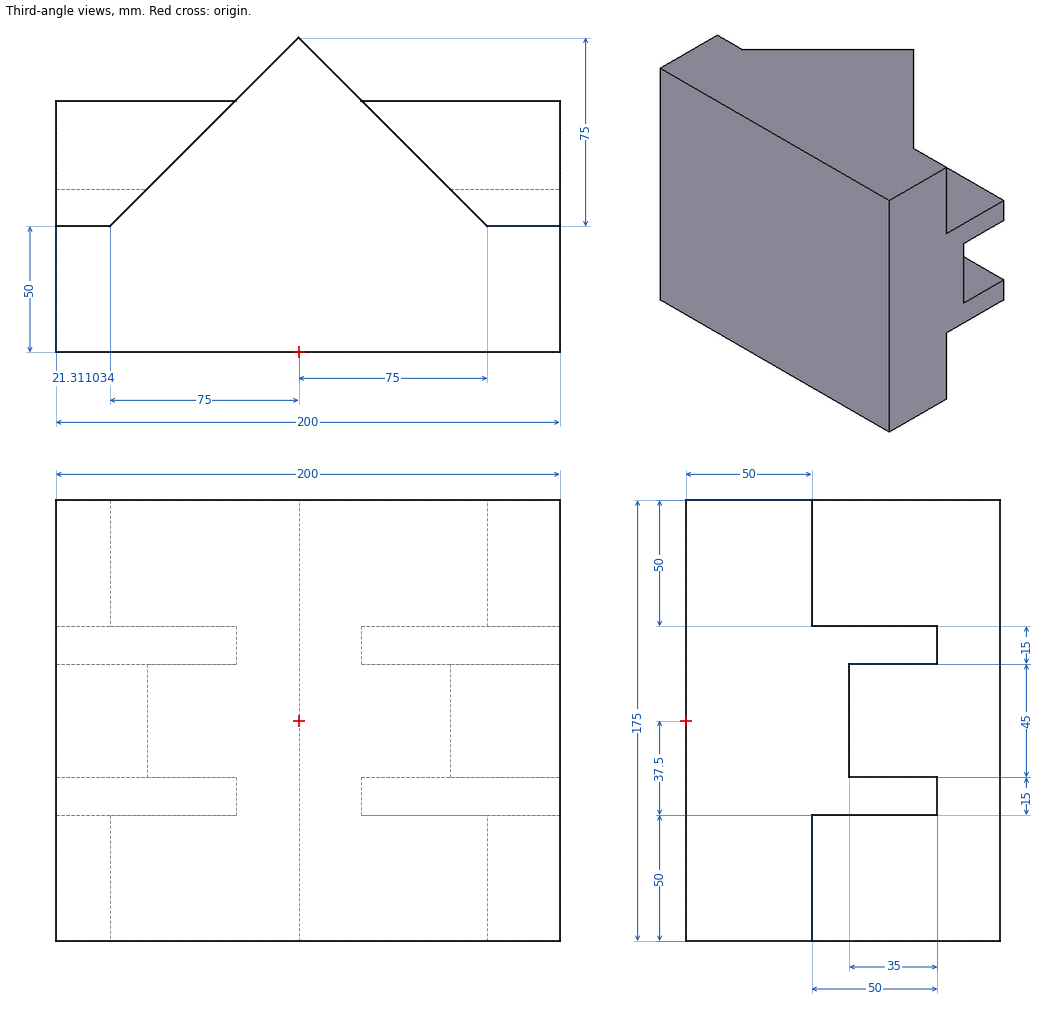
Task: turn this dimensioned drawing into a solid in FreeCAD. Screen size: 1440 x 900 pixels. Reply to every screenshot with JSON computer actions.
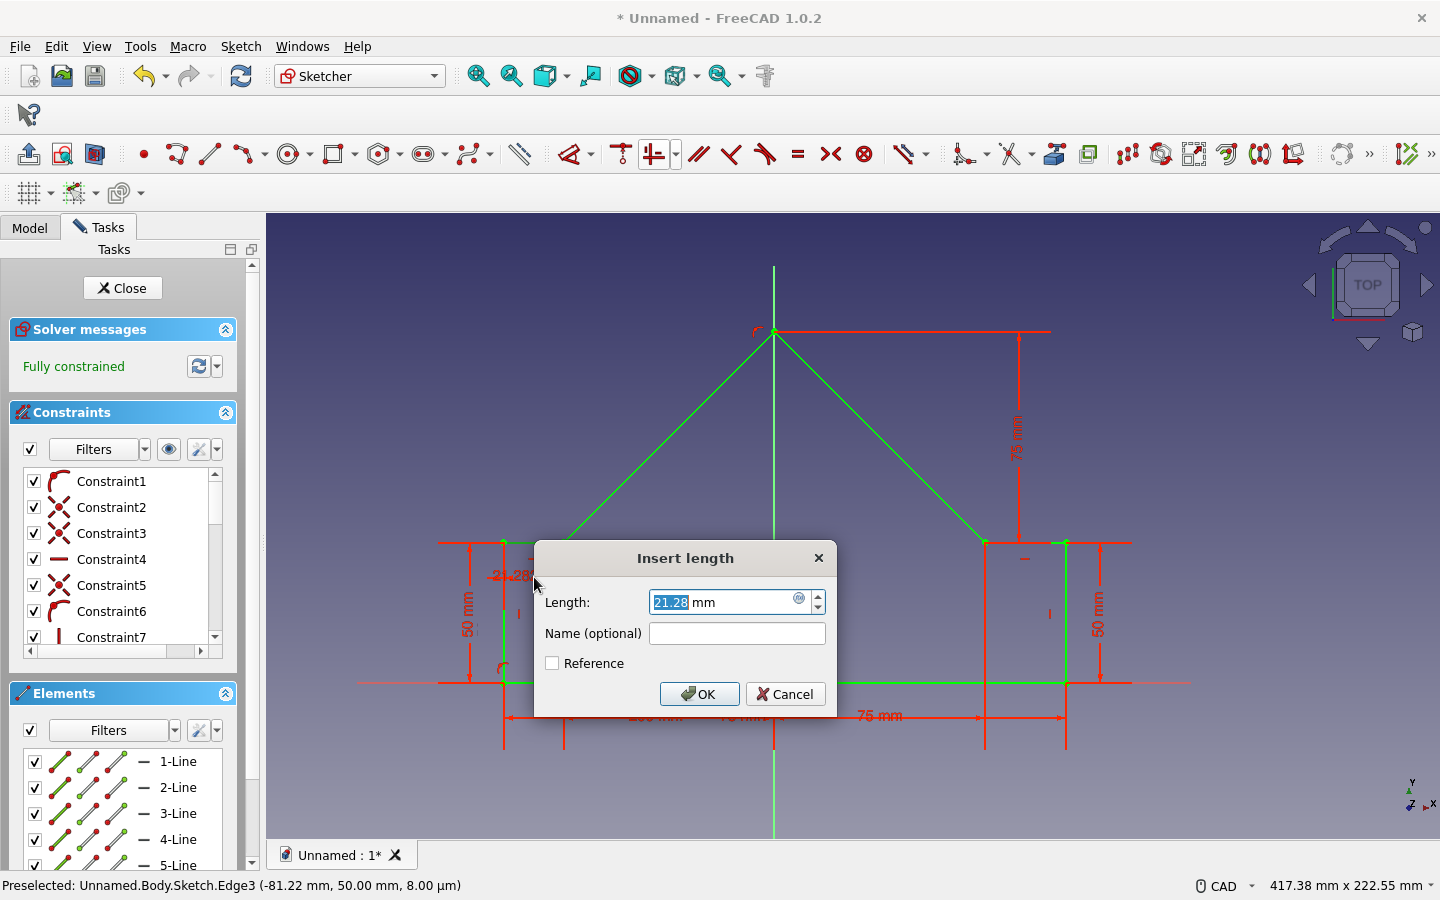
{"action": "type", "text": "21.311034"}
{"action": "key", "text": "Return"}
{"action": "key", "text": "Escape"}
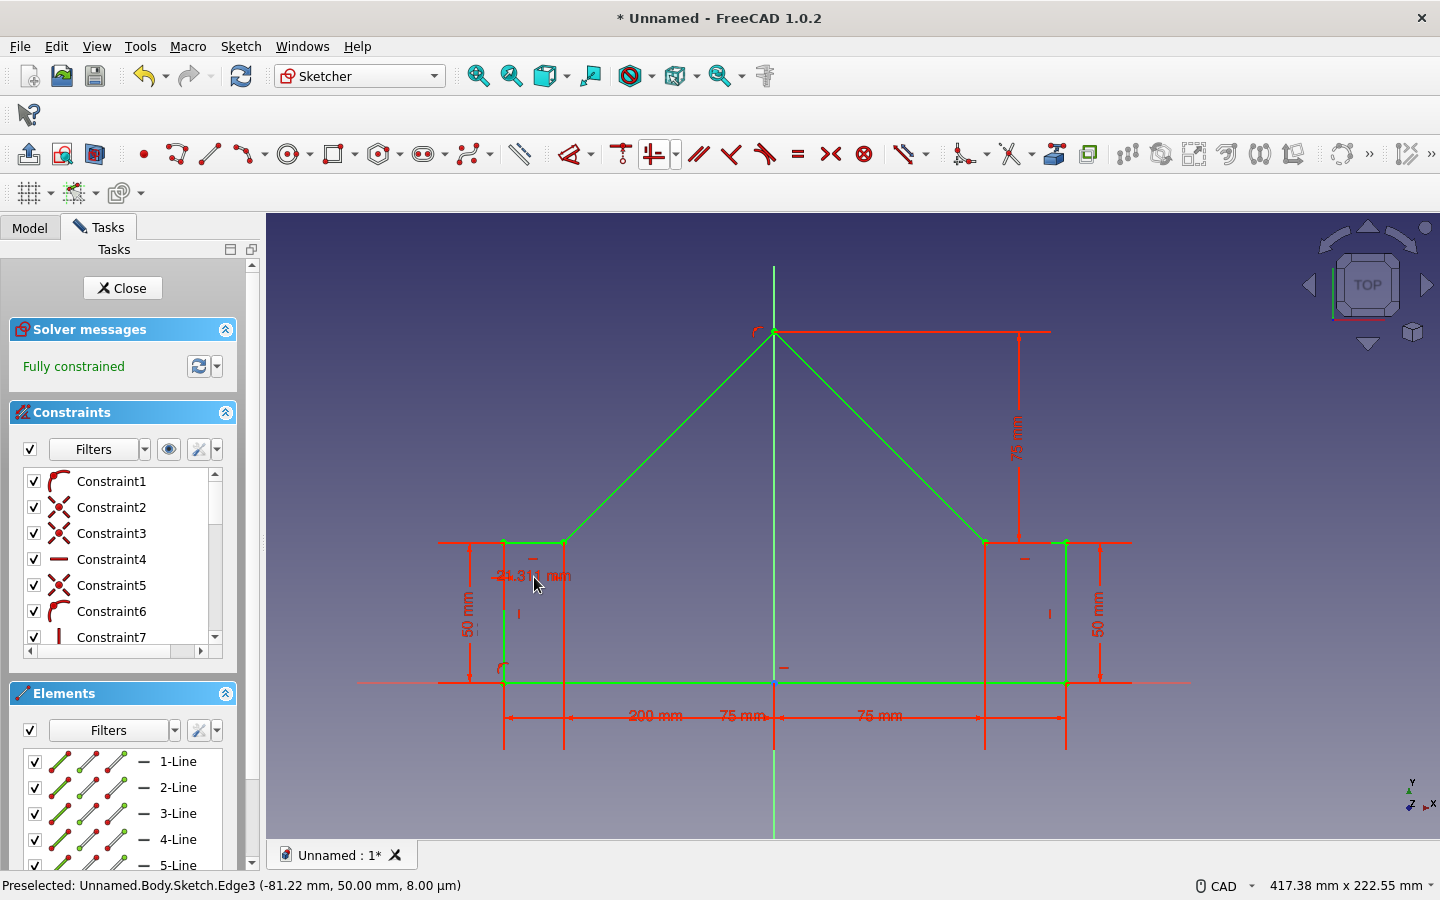
{"action": "left_click", "coordinate": [123, 288]}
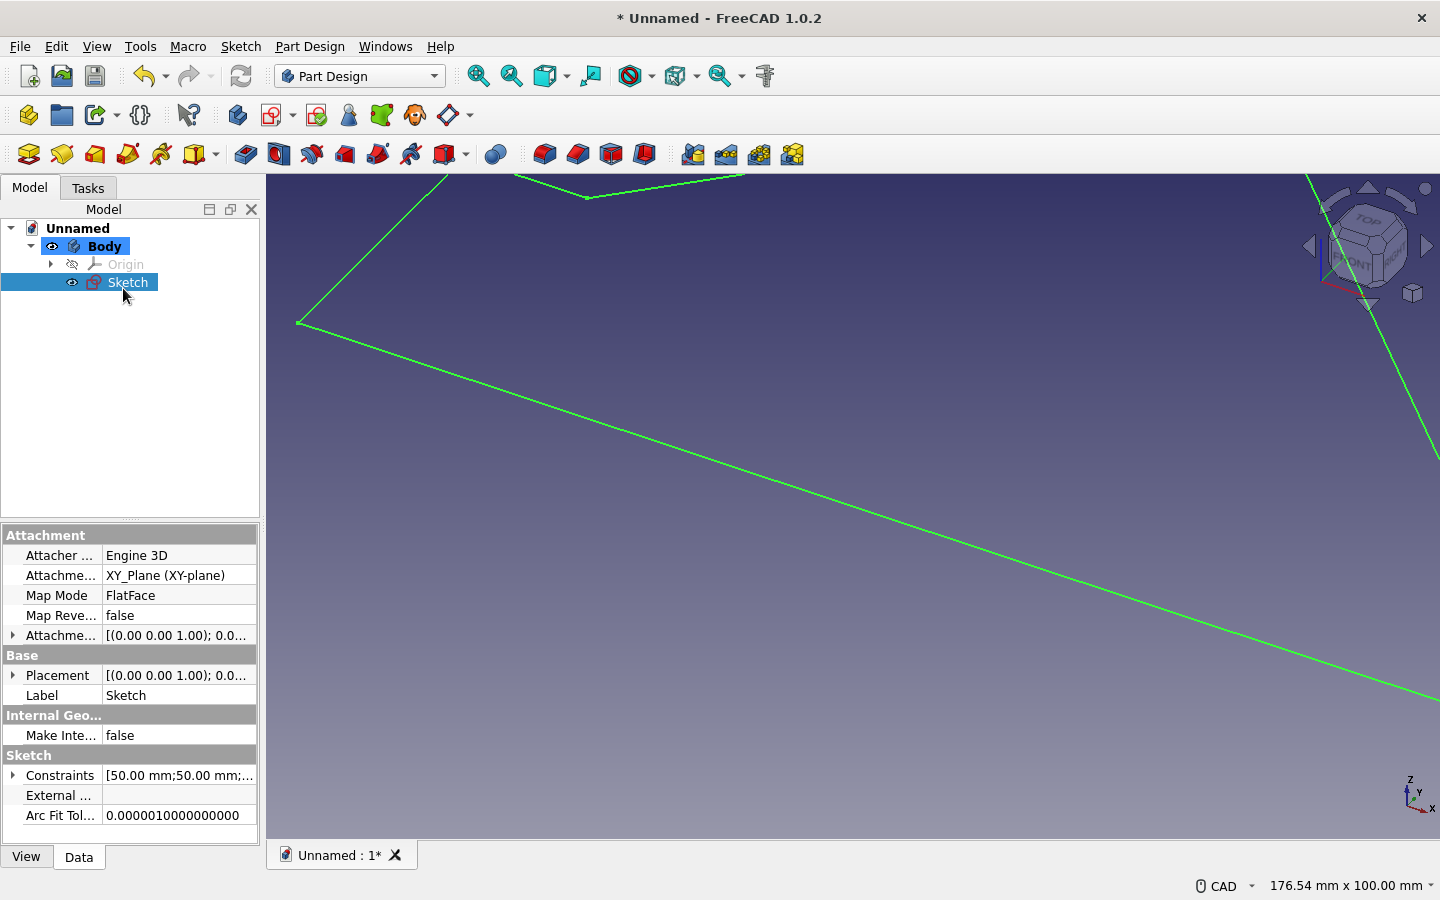
{"action": "left_click", "coordinate": [29, 154]}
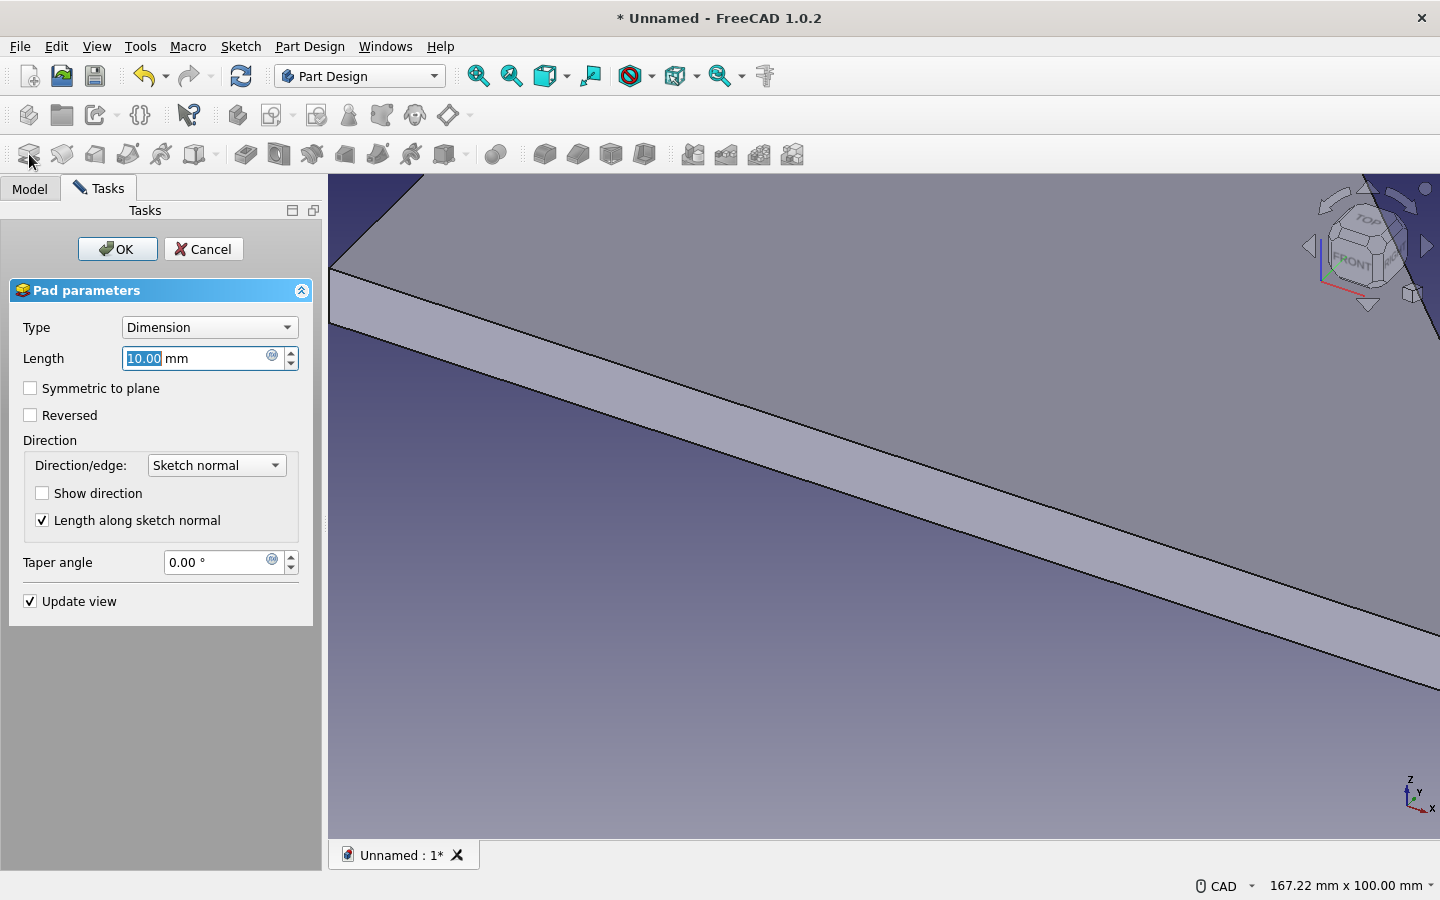
{"action": "type", "text": "175"}
{"action": "key", "text": "Tab"}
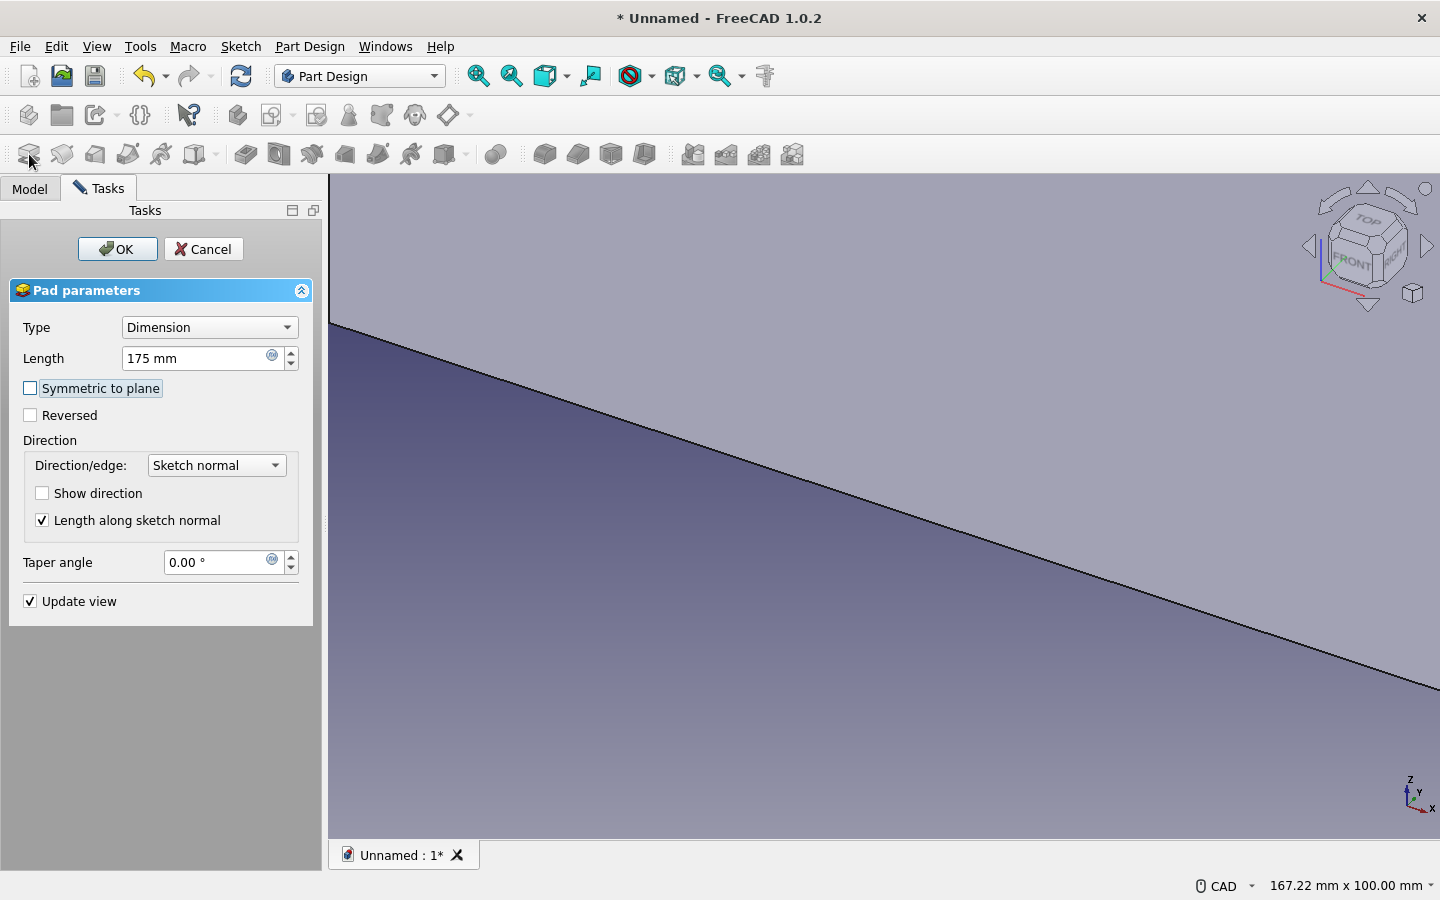
{"action": "left_click", "coordinate": [31, 388]}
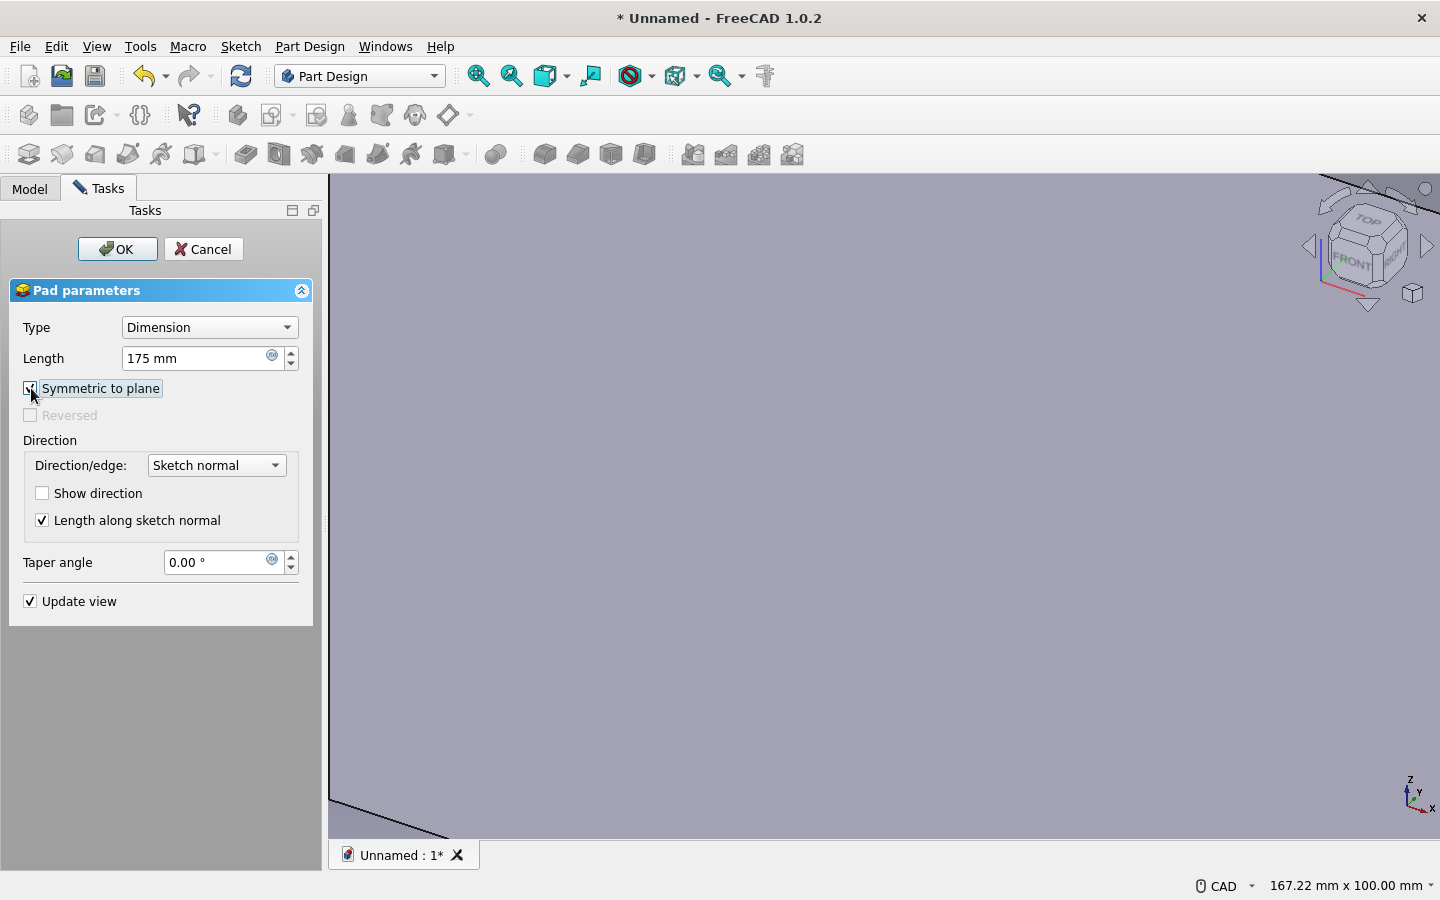
{"action": "left_click", "coordinate": [118, 249]}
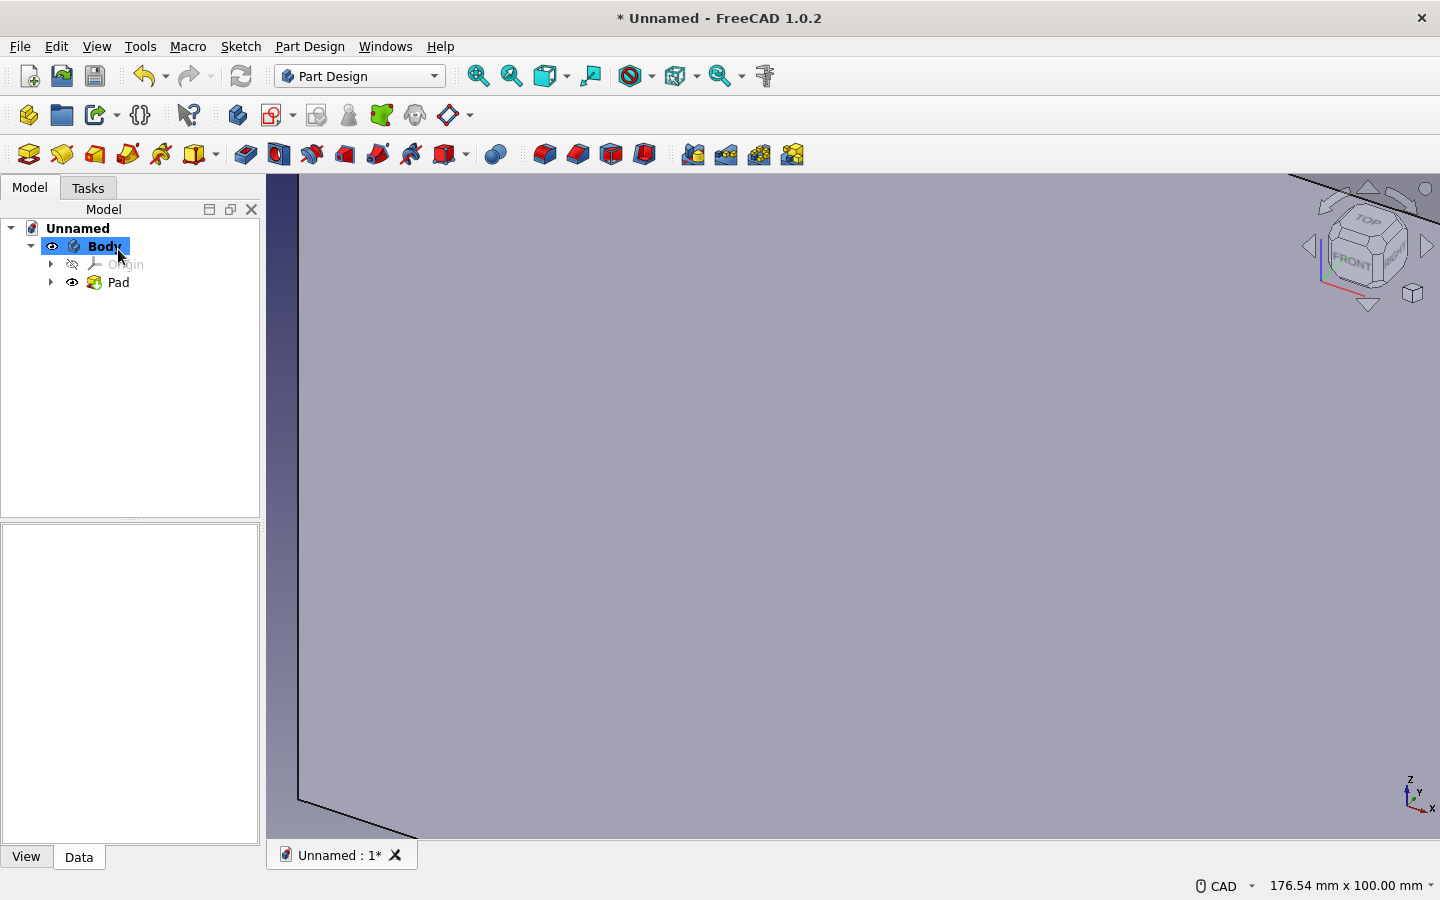
{"action": "left_click", "coordinate": [479, 76]}